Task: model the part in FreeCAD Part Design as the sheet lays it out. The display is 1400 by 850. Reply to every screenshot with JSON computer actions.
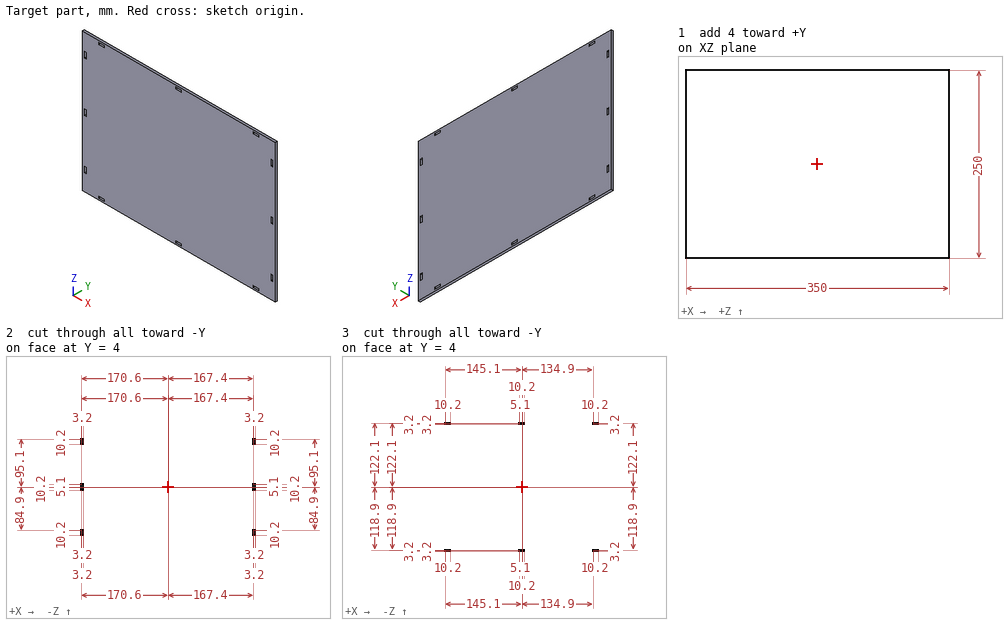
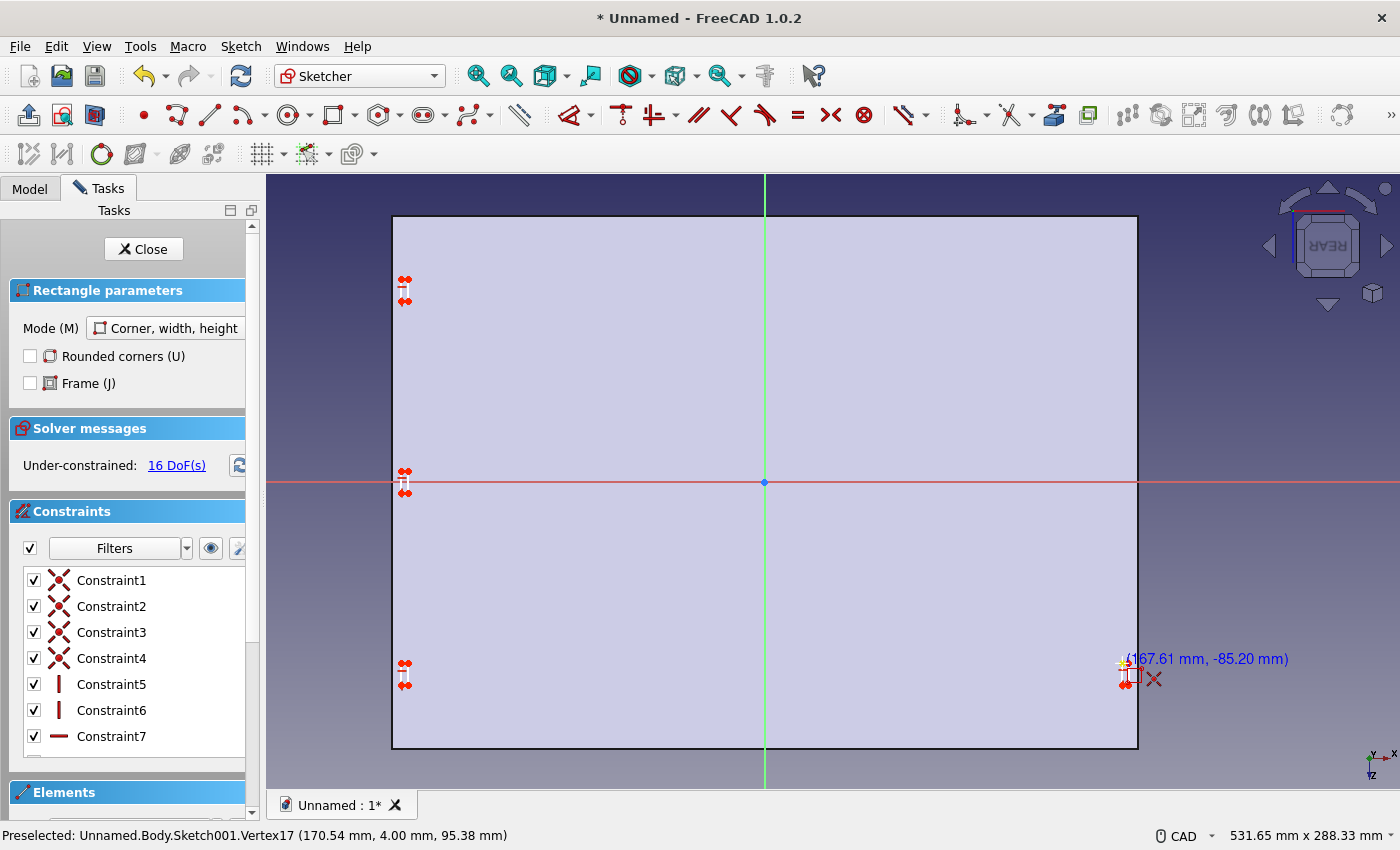
{"action": "scroll", "coordinate": [1122, 471], "scroll_direction": "up", "scroll_amount": 5}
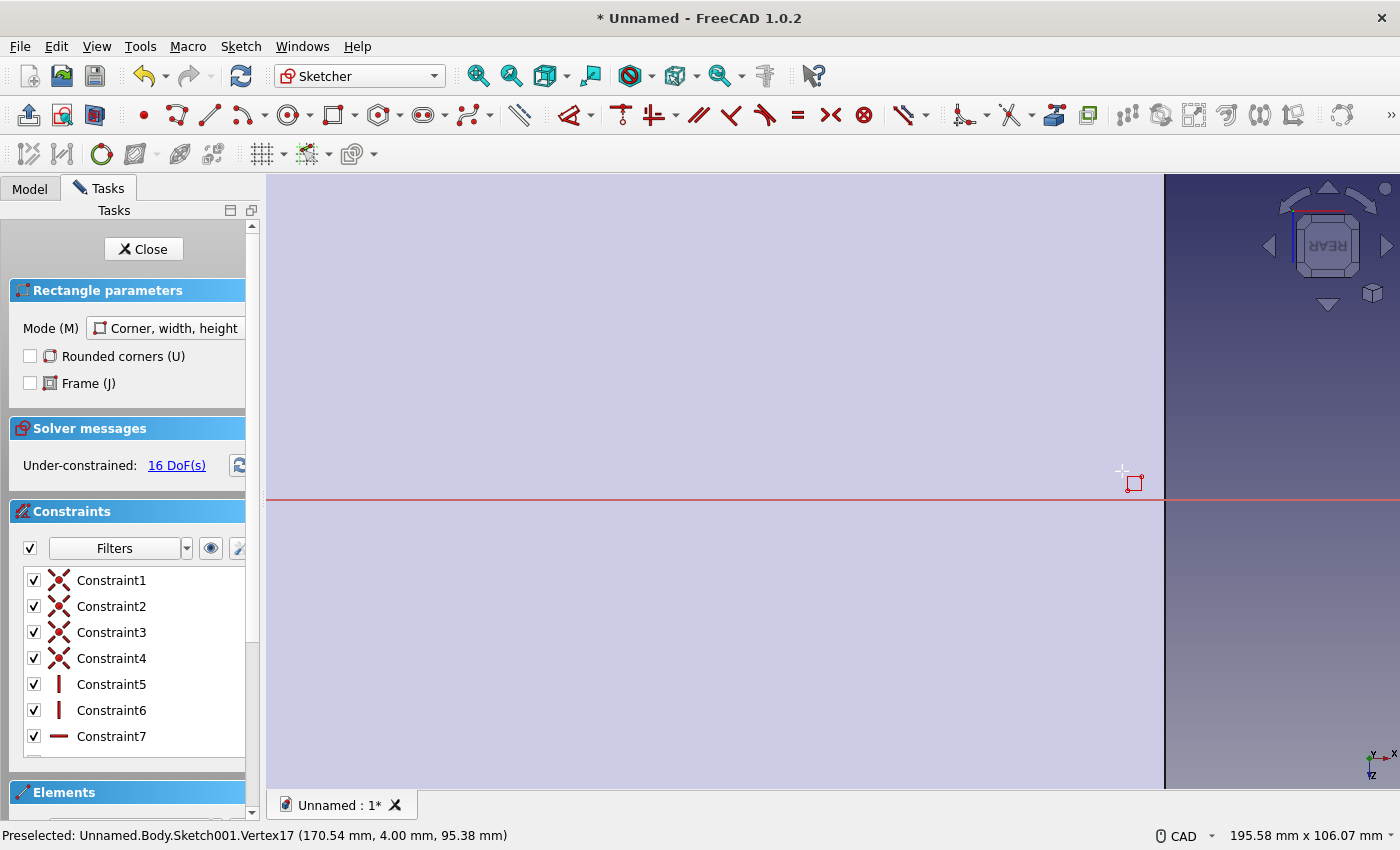
{"action": "left_click", "coordinate": [1121, 471]}
{"action": "left_click", "coordinate": [1139, 530]}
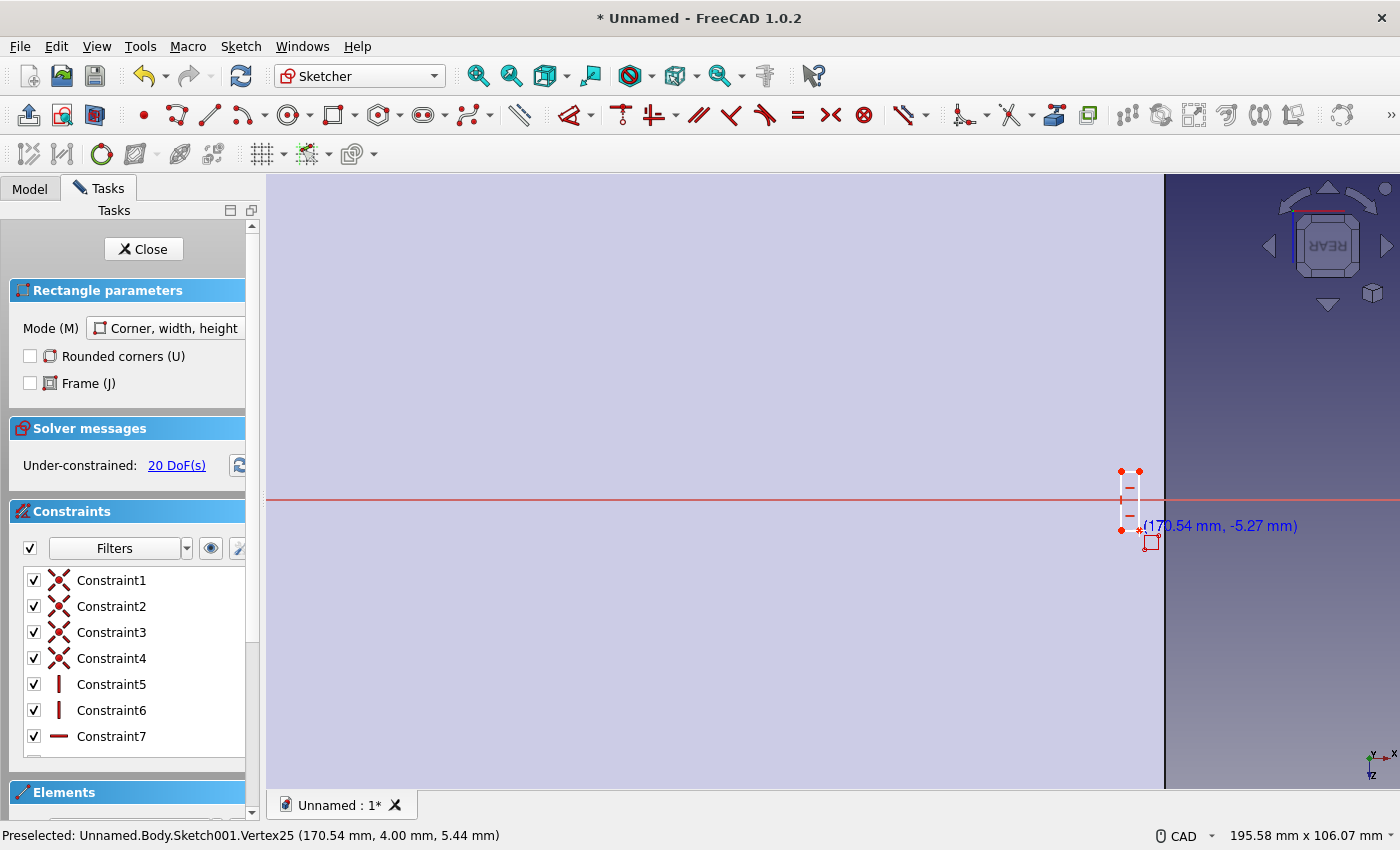
{"action": "scroll", "coordinate": [1122, 470], "scroll_direction": "down", "scroll_amount": 5}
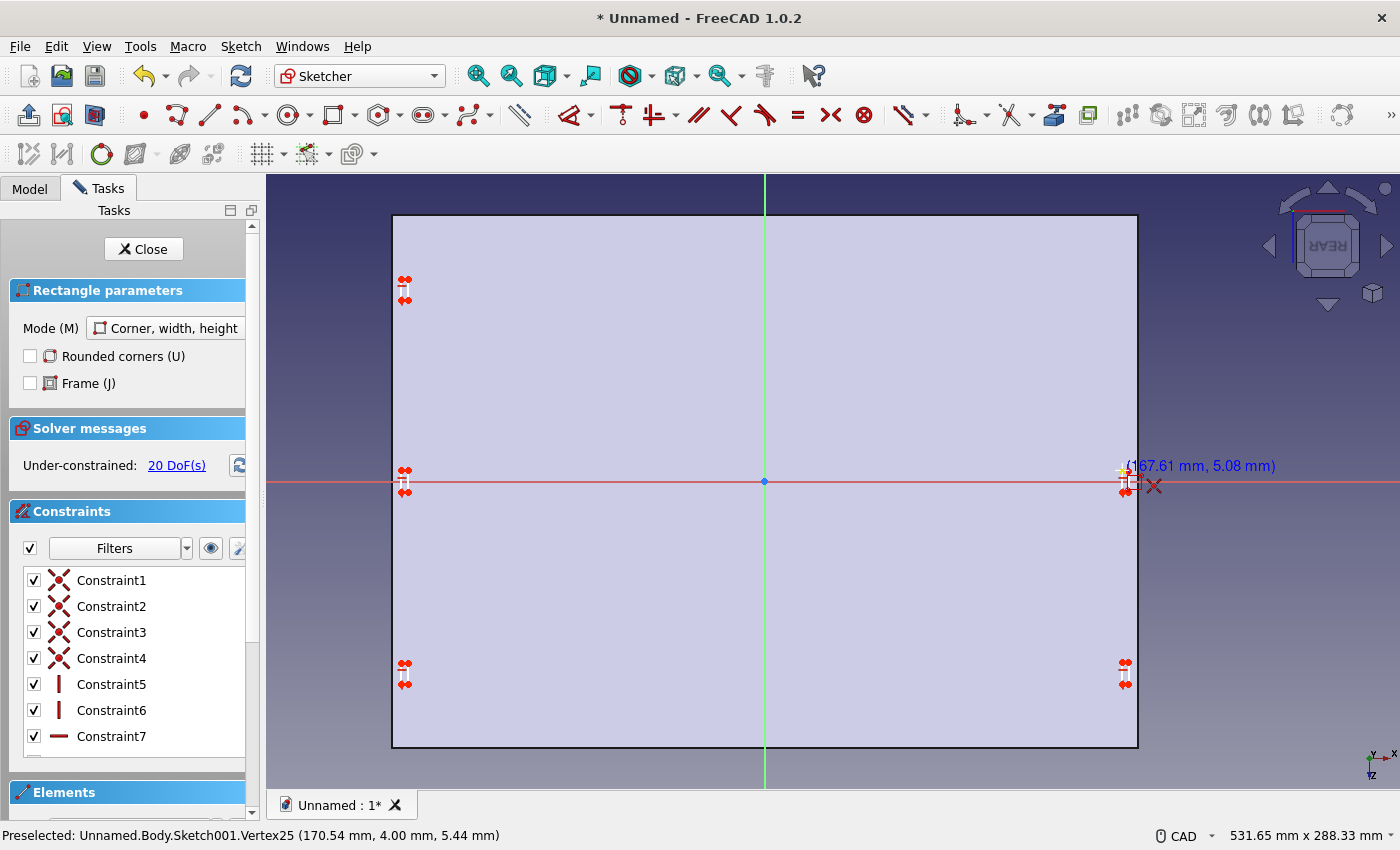
{"action": "scroll", "coordinate": [1122, 279], "scroll_direction": "up", "scroll_amount": 5}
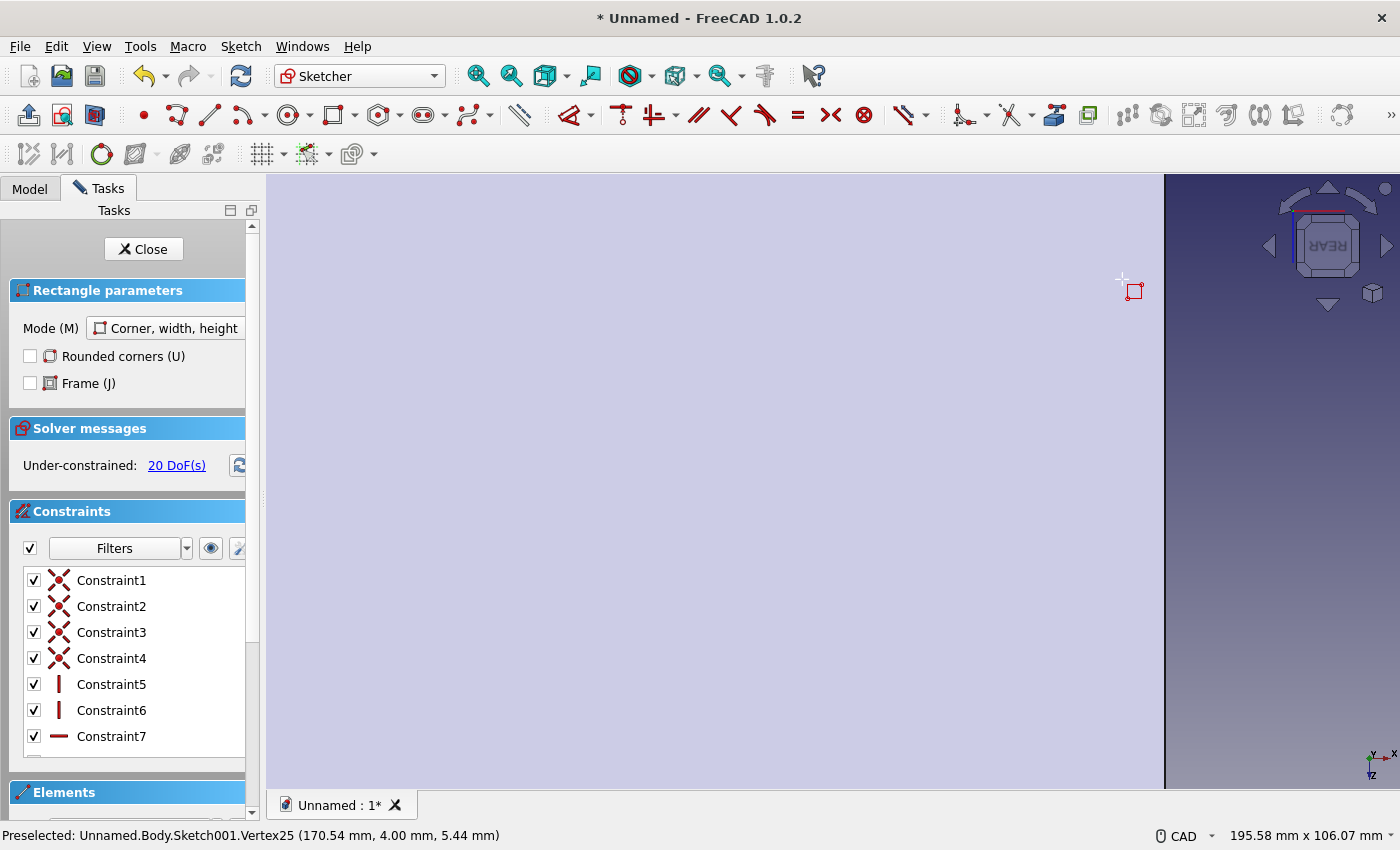
{"action": "left_click", "coordinate": [1121, 278]}
{"action": "left_click", "coordinate": [1139, 337]}
{"action": "key", "text": "Escape"}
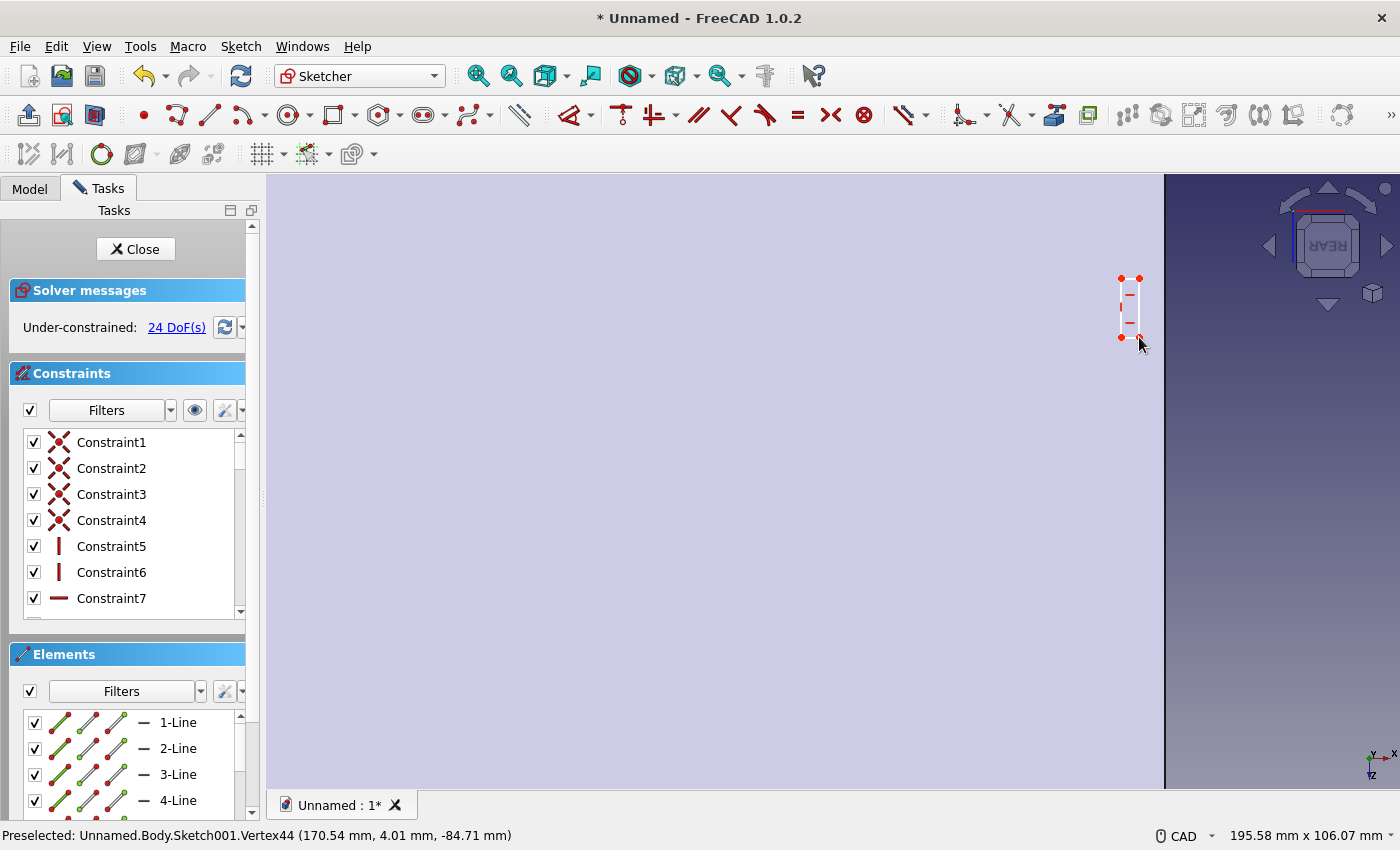
{"action": "left_click", "coordinate": [568, 116]}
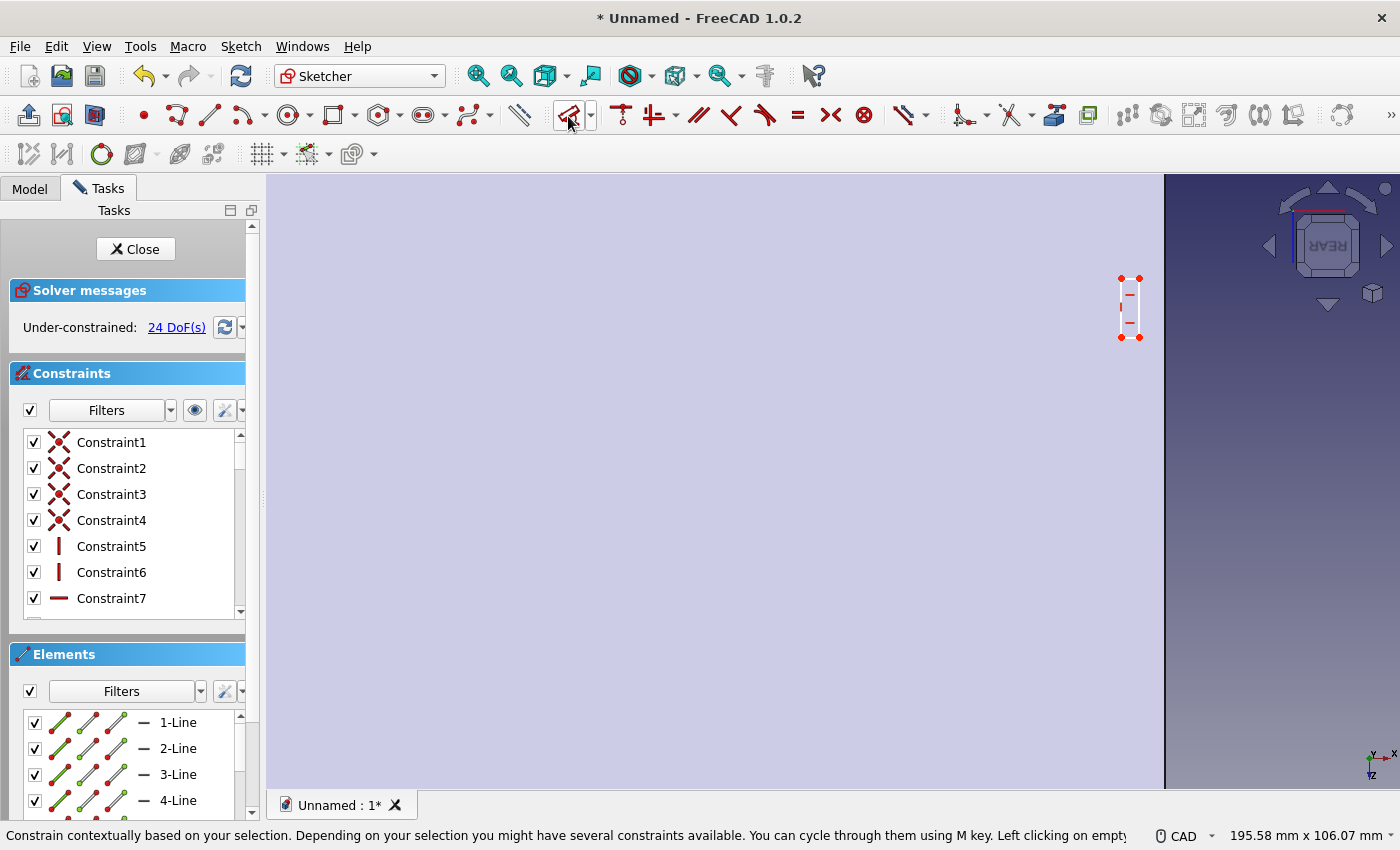
{"action": "scroll", "coordinate": [1122, 279], "scroll_direction": "down", "scroll_amount": 5}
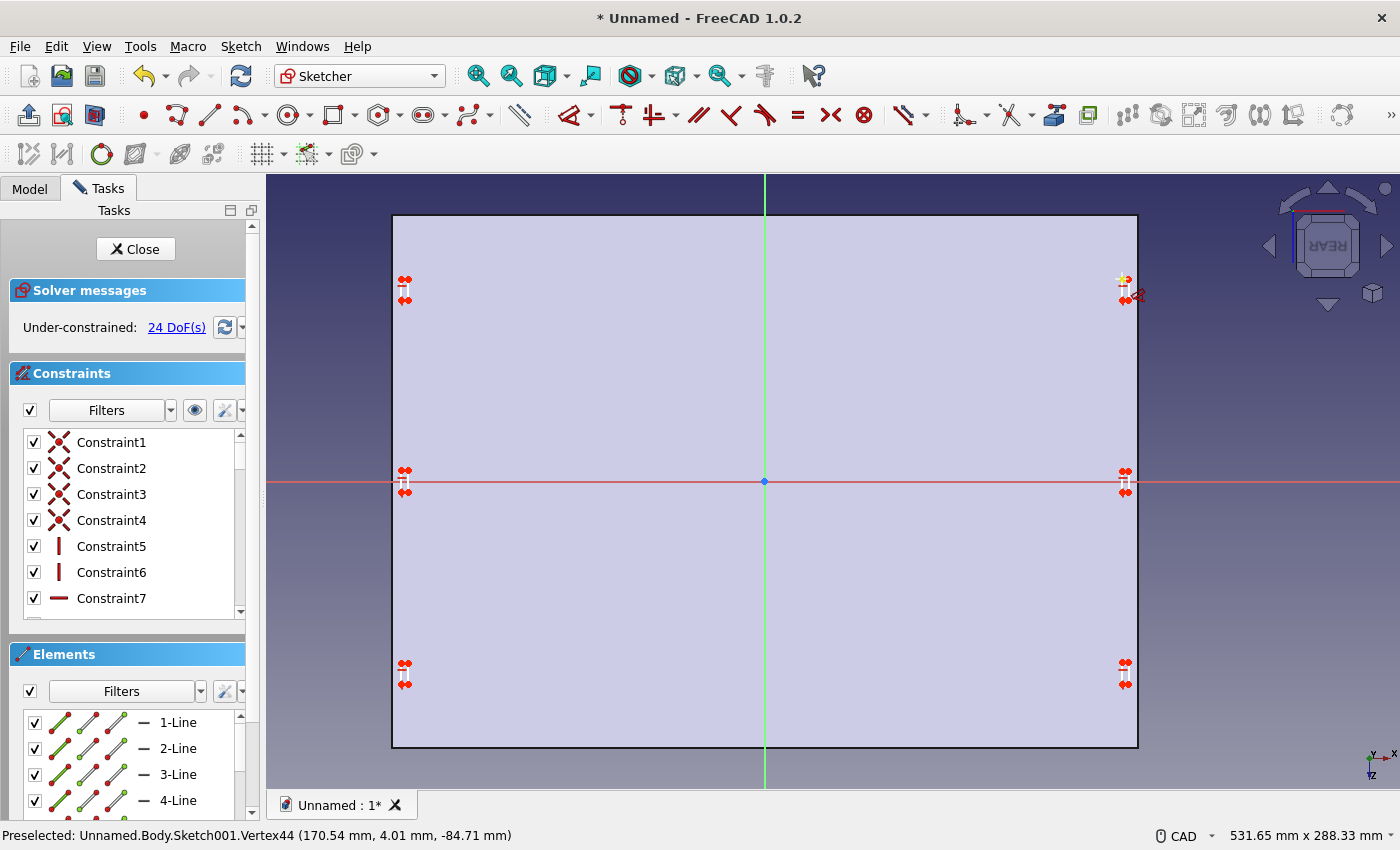
{"action": "scroll", "coordinate": [405, 301], "scroll_direction": "up", "scroll_amount": 9}